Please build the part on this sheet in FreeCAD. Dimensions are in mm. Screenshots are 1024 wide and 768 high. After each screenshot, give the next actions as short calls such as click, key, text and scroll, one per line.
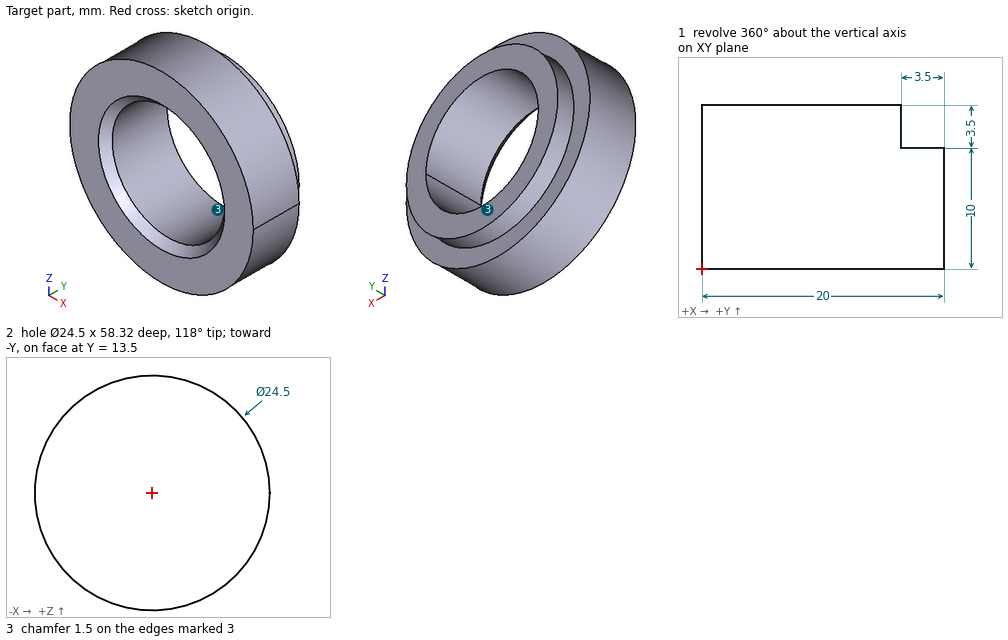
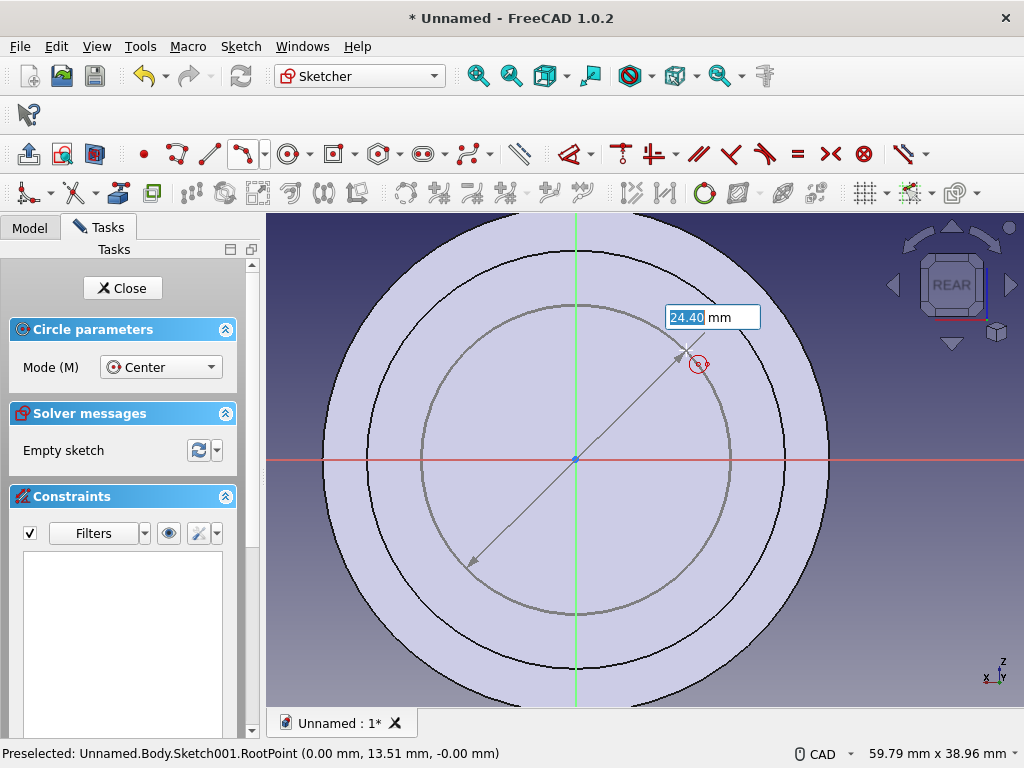
text(24.5)
key(Return)
key(Escape)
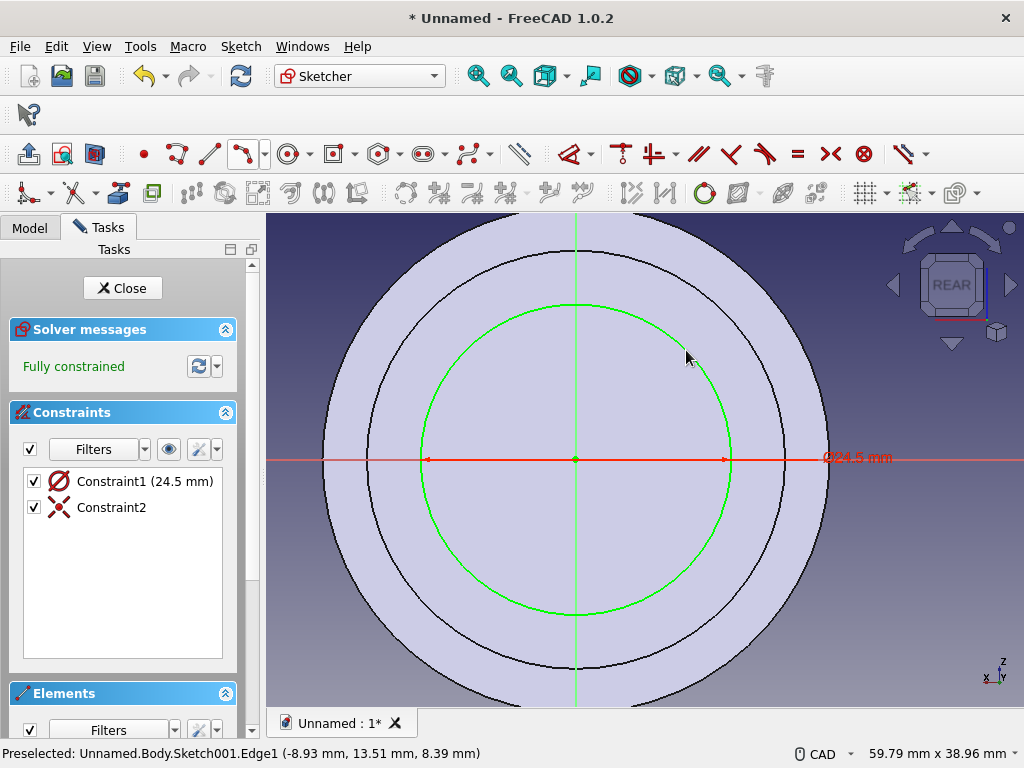
click(123, 288)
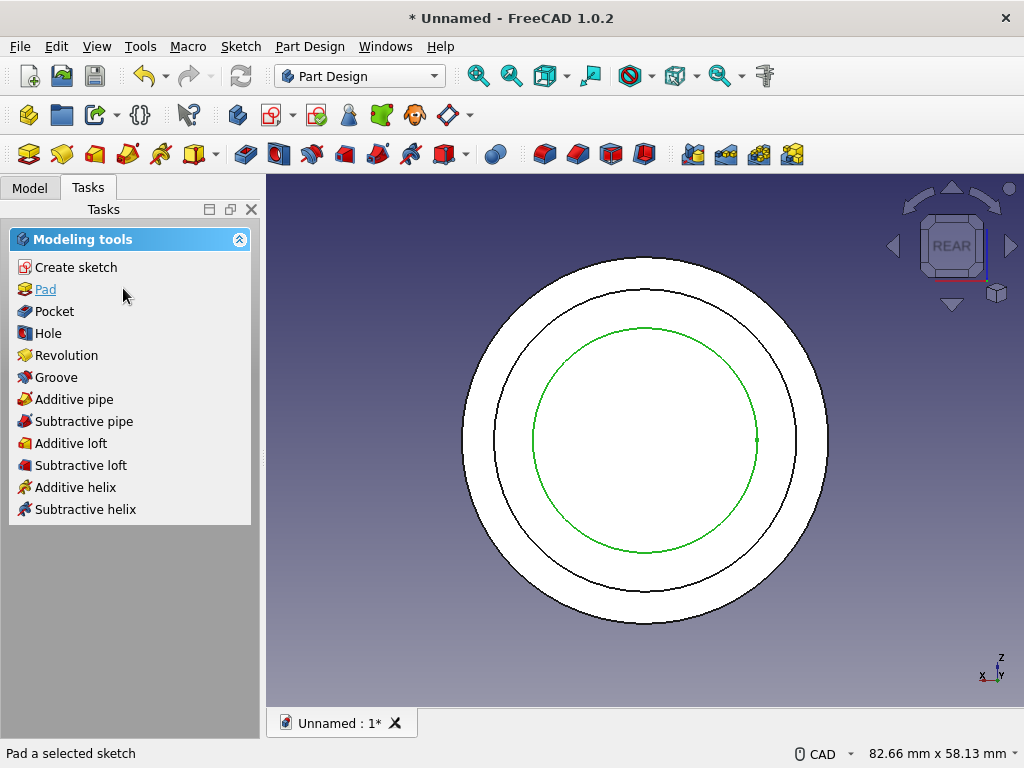
click(279, 154)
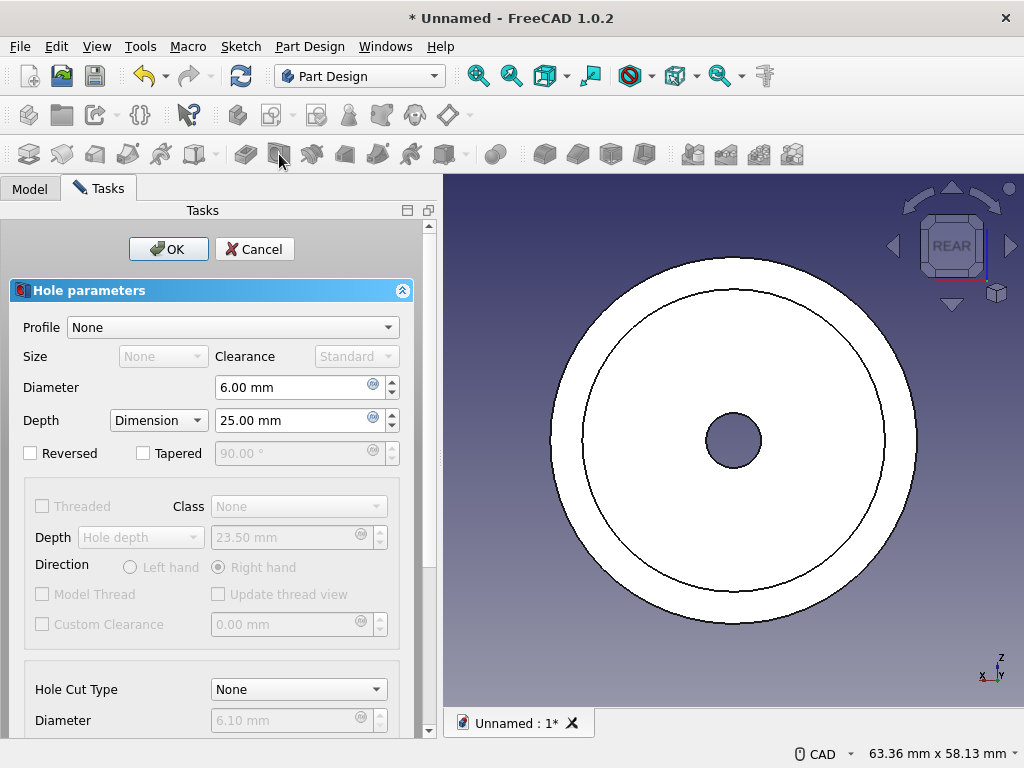
triple_click(300, 388)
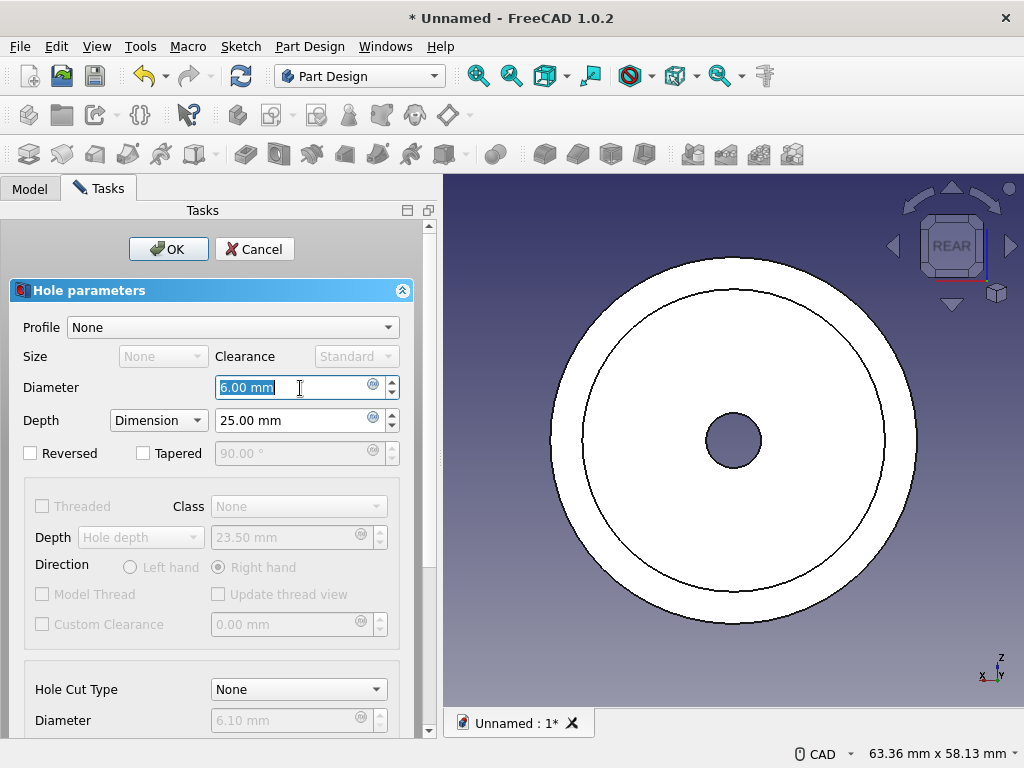
text(24.5)
key(Tab)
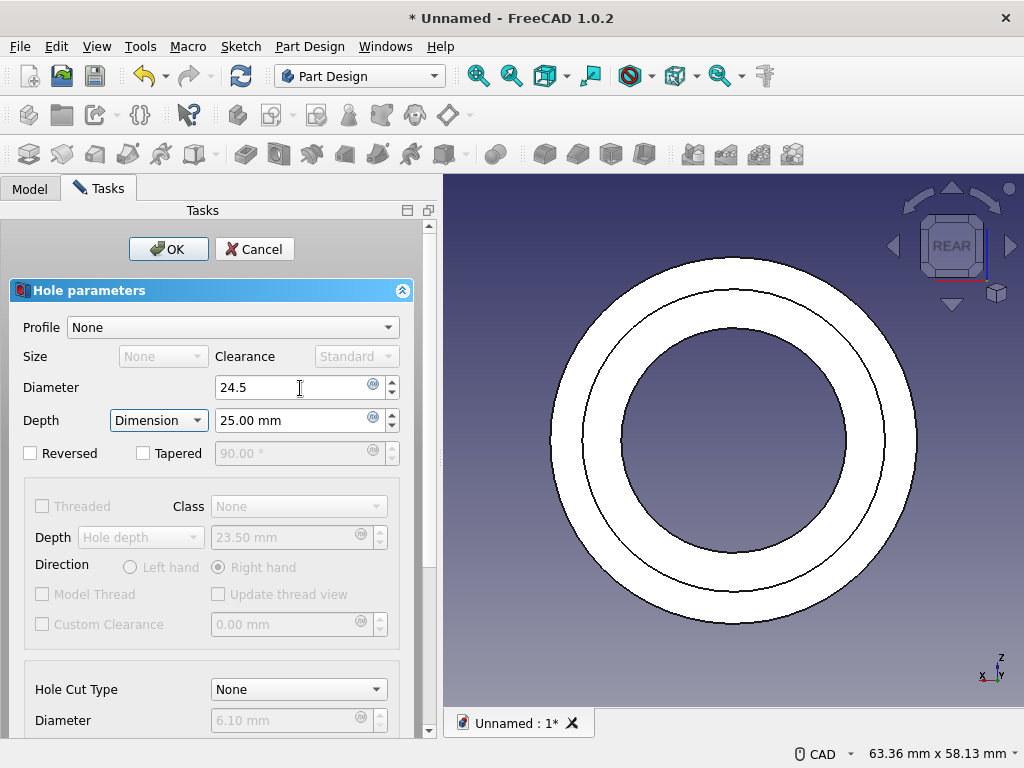
triple_click(300, 420)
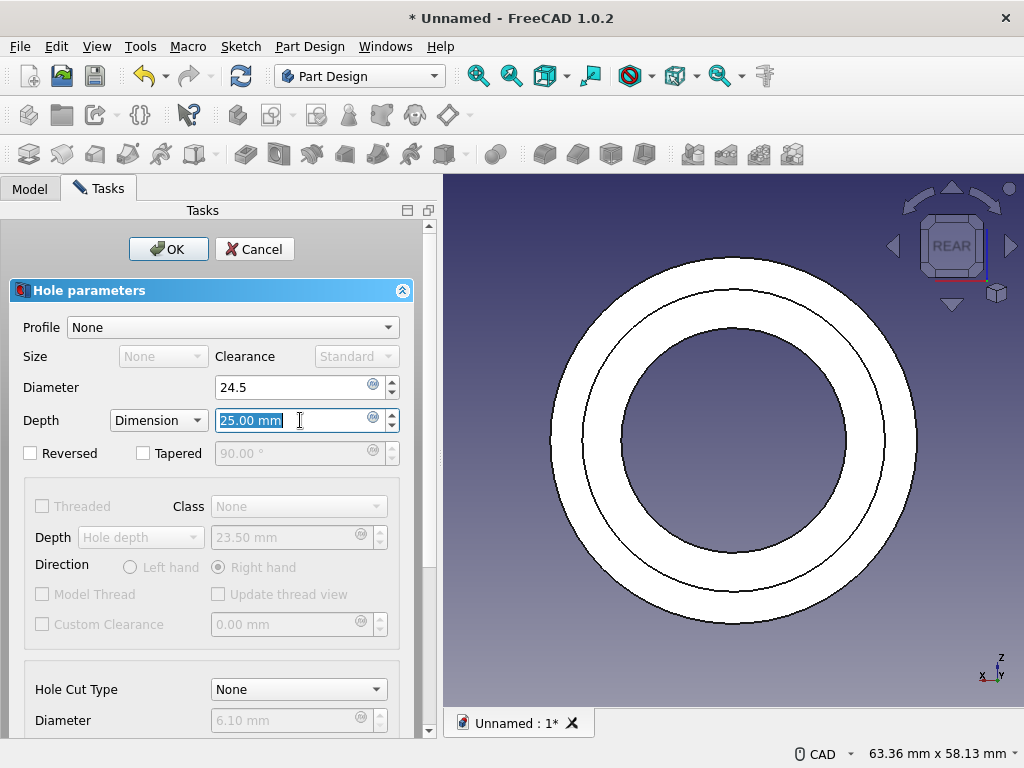
text(58.32)
key(Tab)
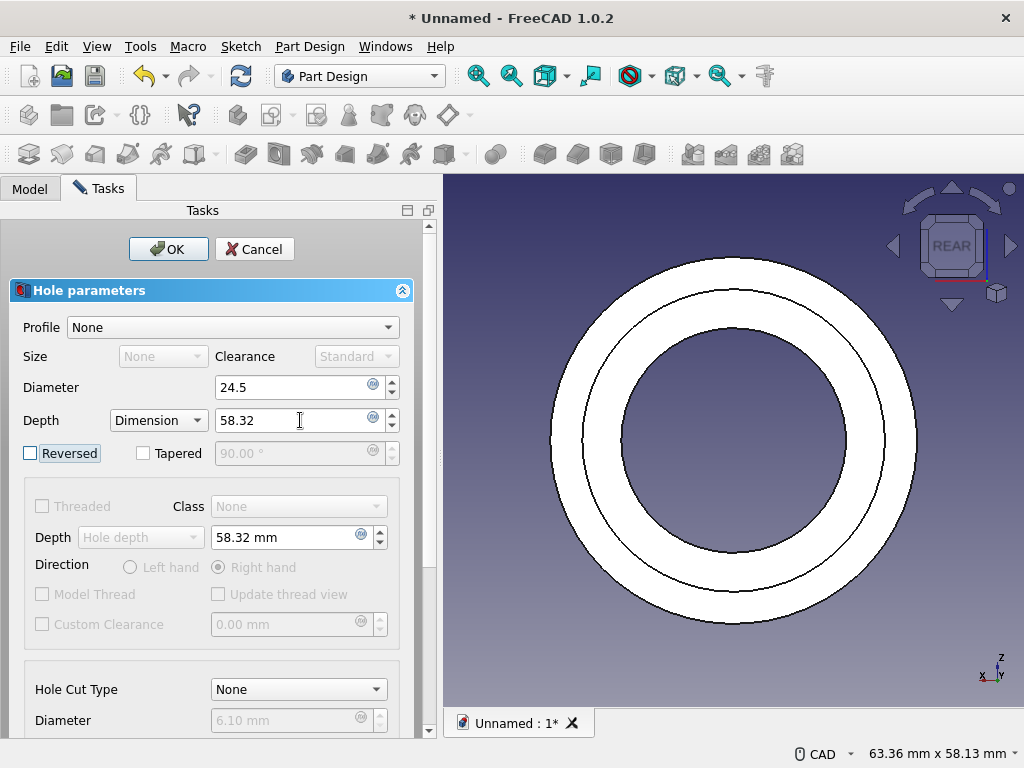
click(169, 249)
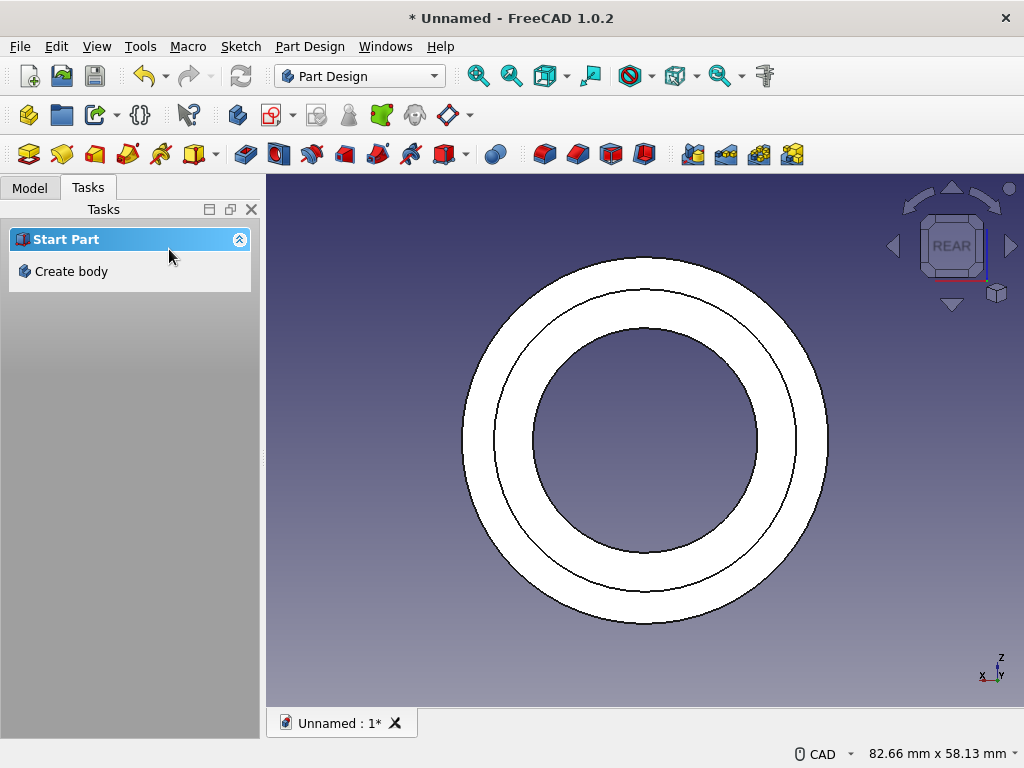
key(0)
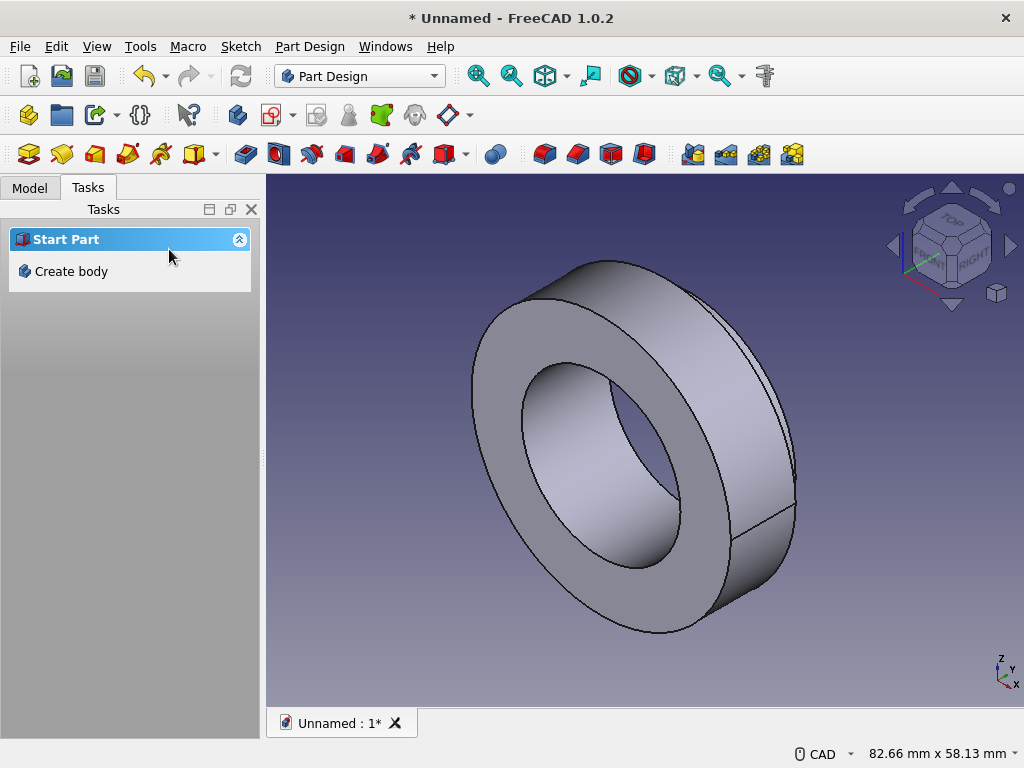
click(522, 419)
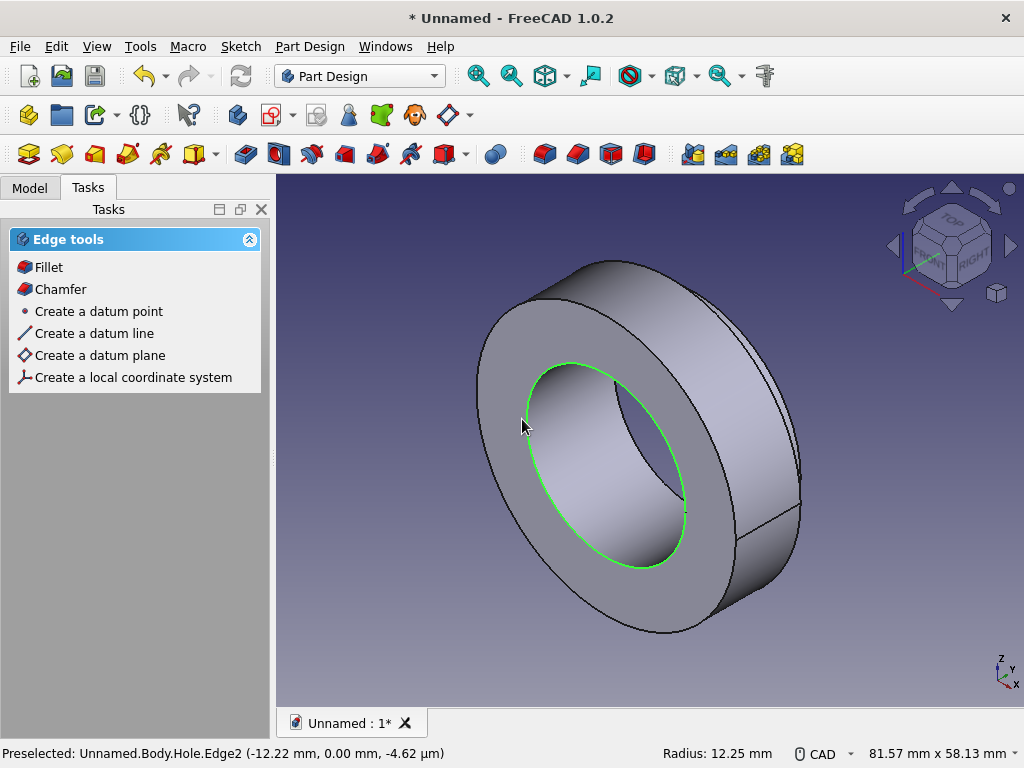
click(578, 154)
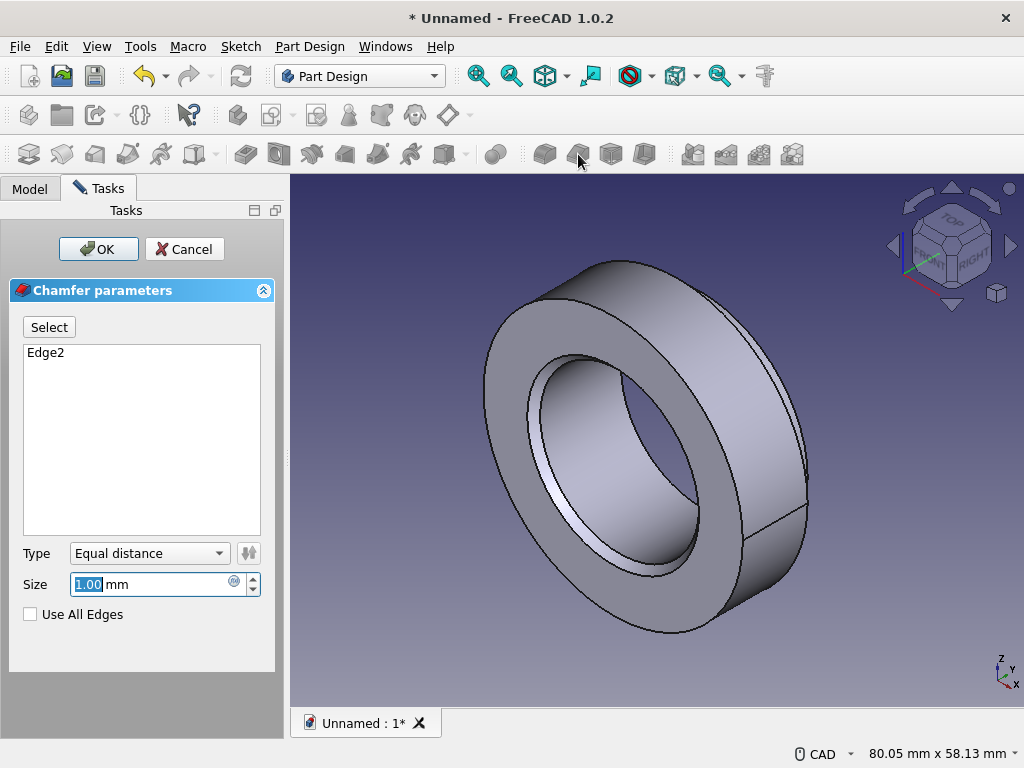
text(1.5)
key(Tab)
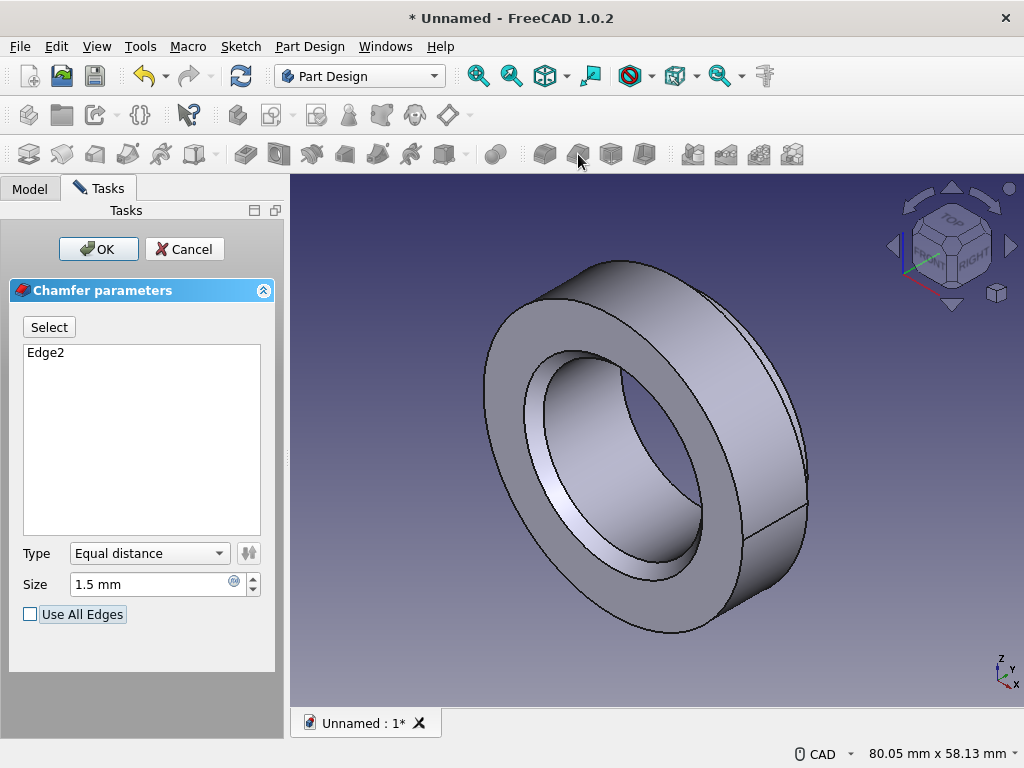
click(99, 249)